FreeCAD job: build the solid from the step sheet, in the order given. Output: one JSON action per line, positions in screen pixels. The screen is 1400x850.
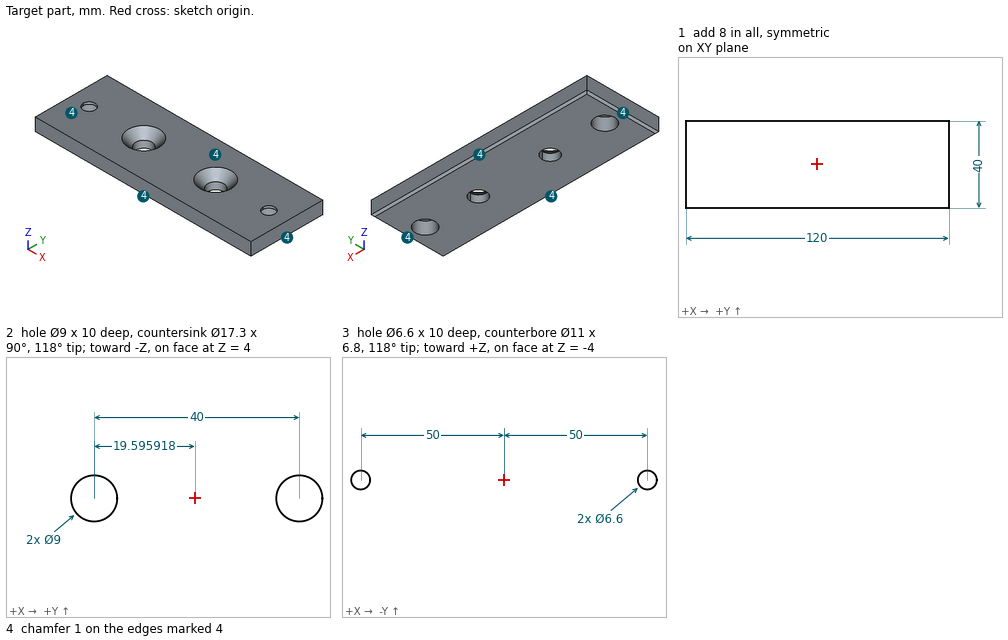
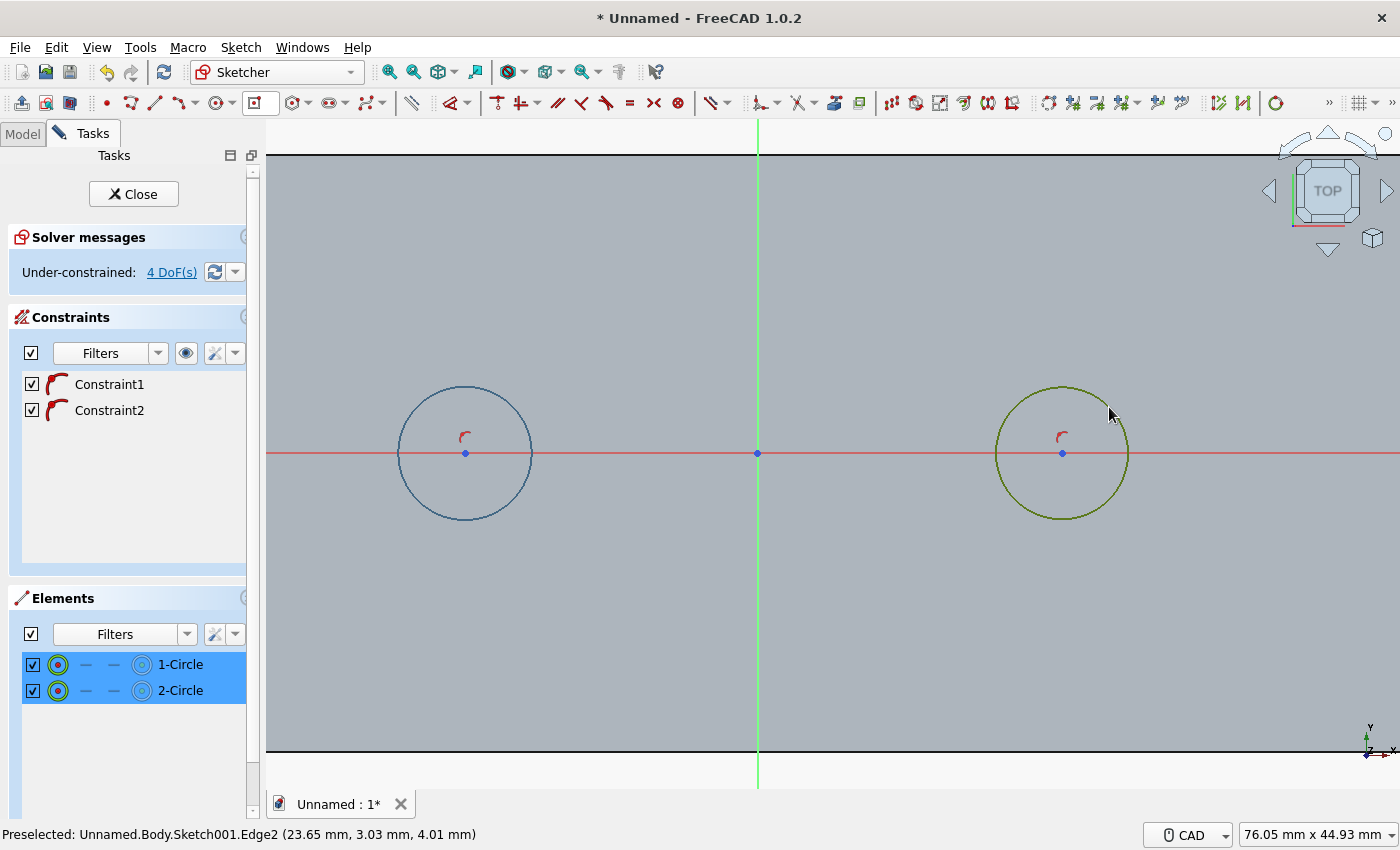
{"action": "key", "text": "e"}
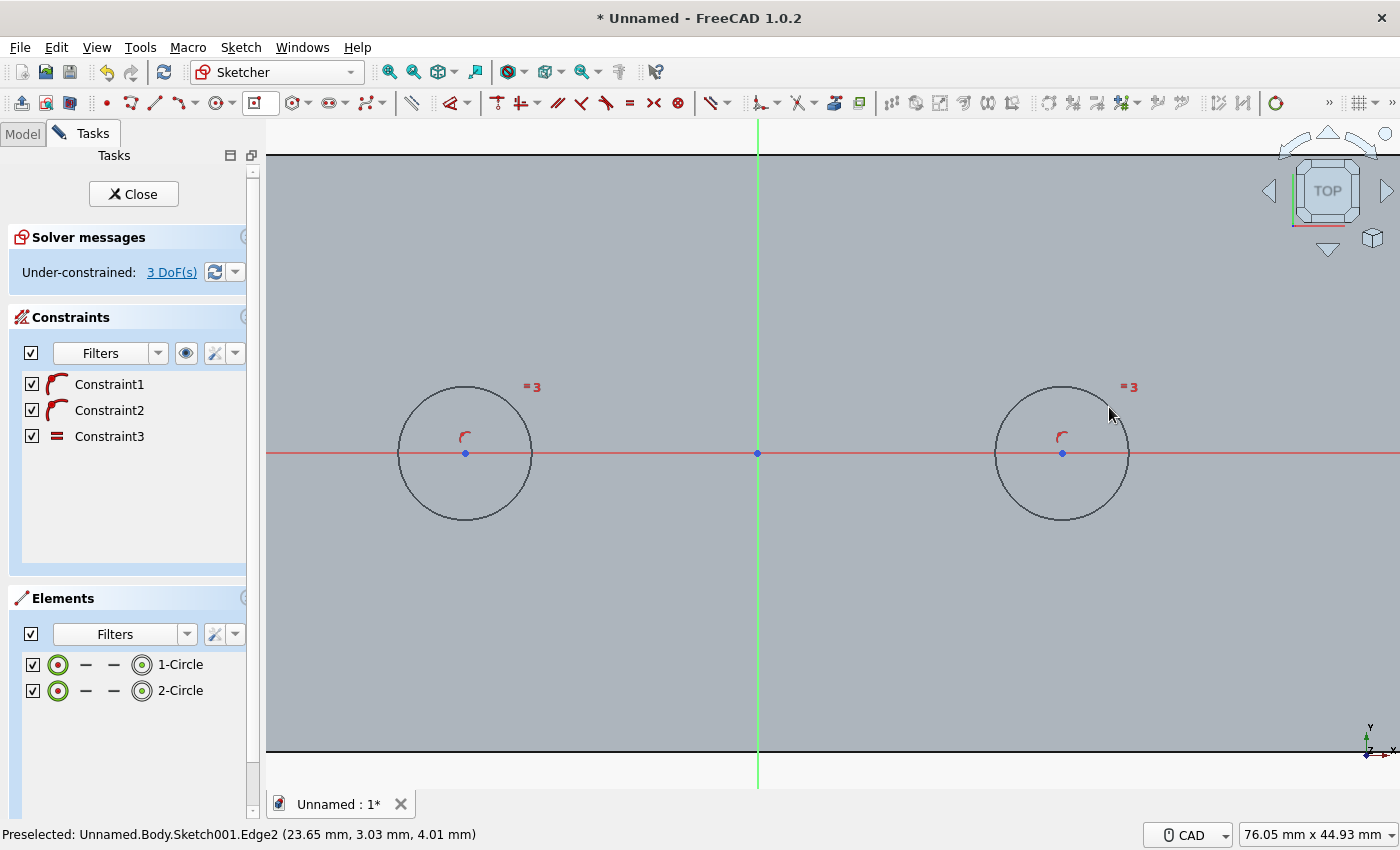
{"action": "left_click", "coordinate": [512, 406]}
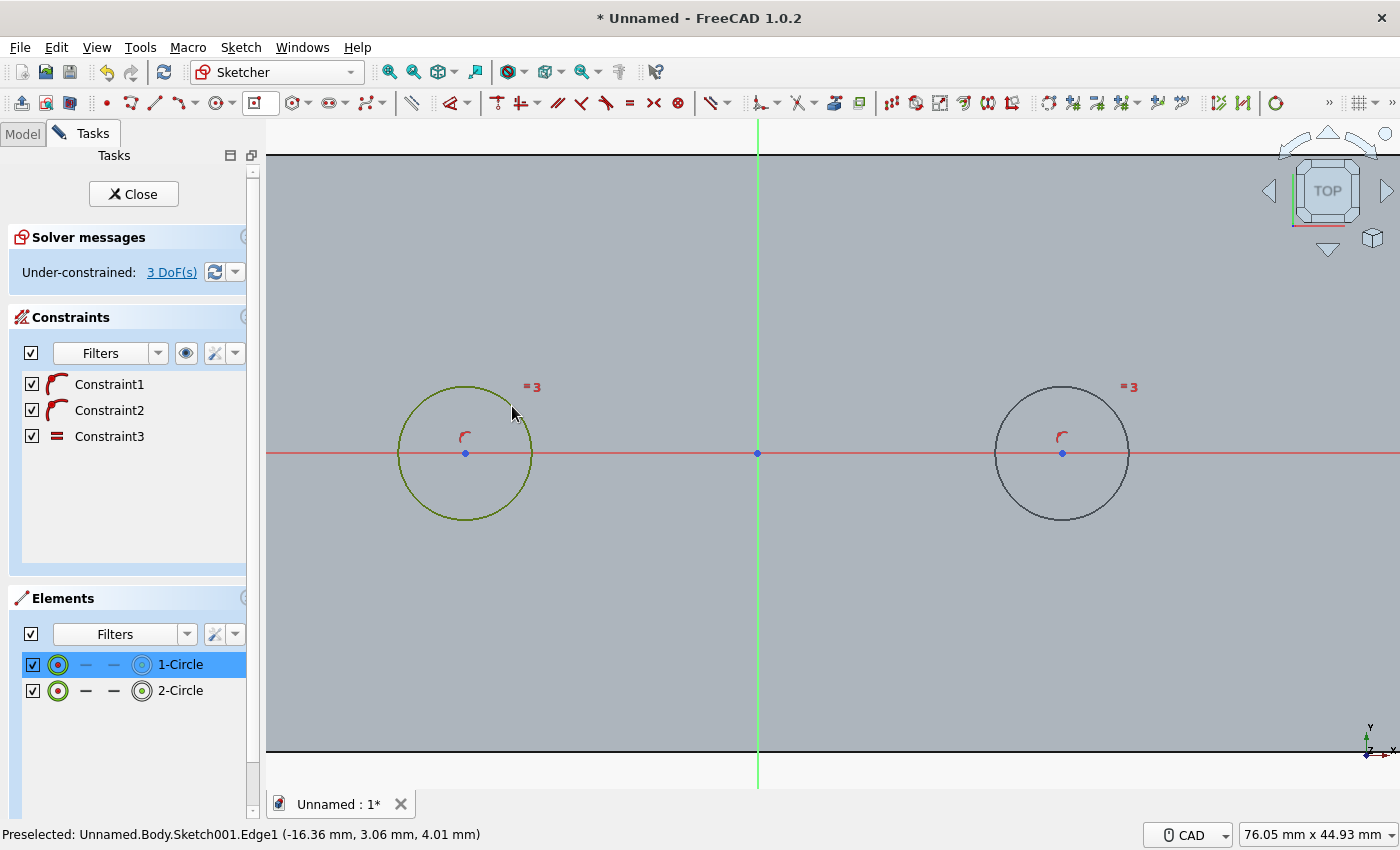
{"action": "key", "text": "k o"}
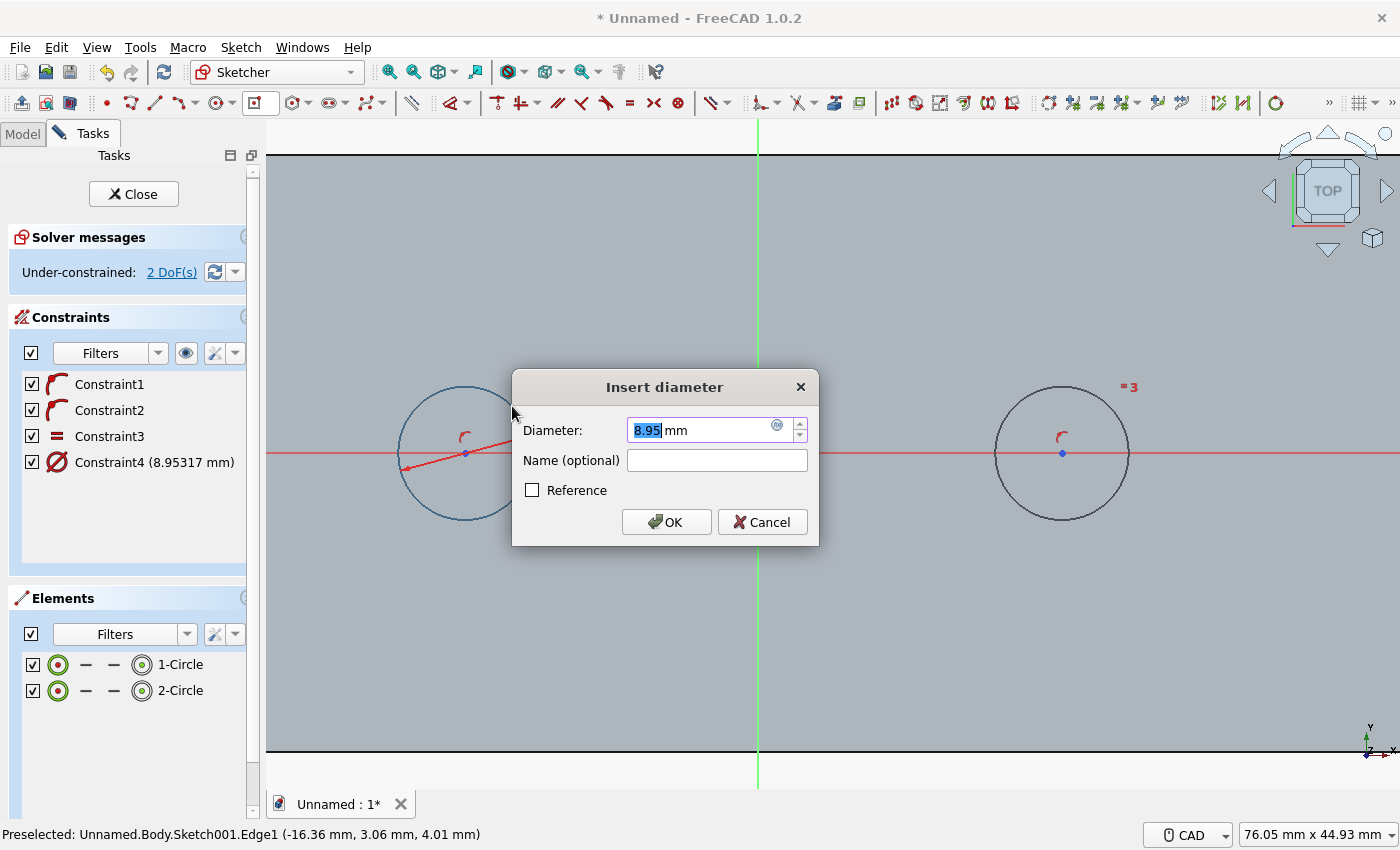
{"action": "type", "text": "9"}
{"action": "key", "text": "Return"}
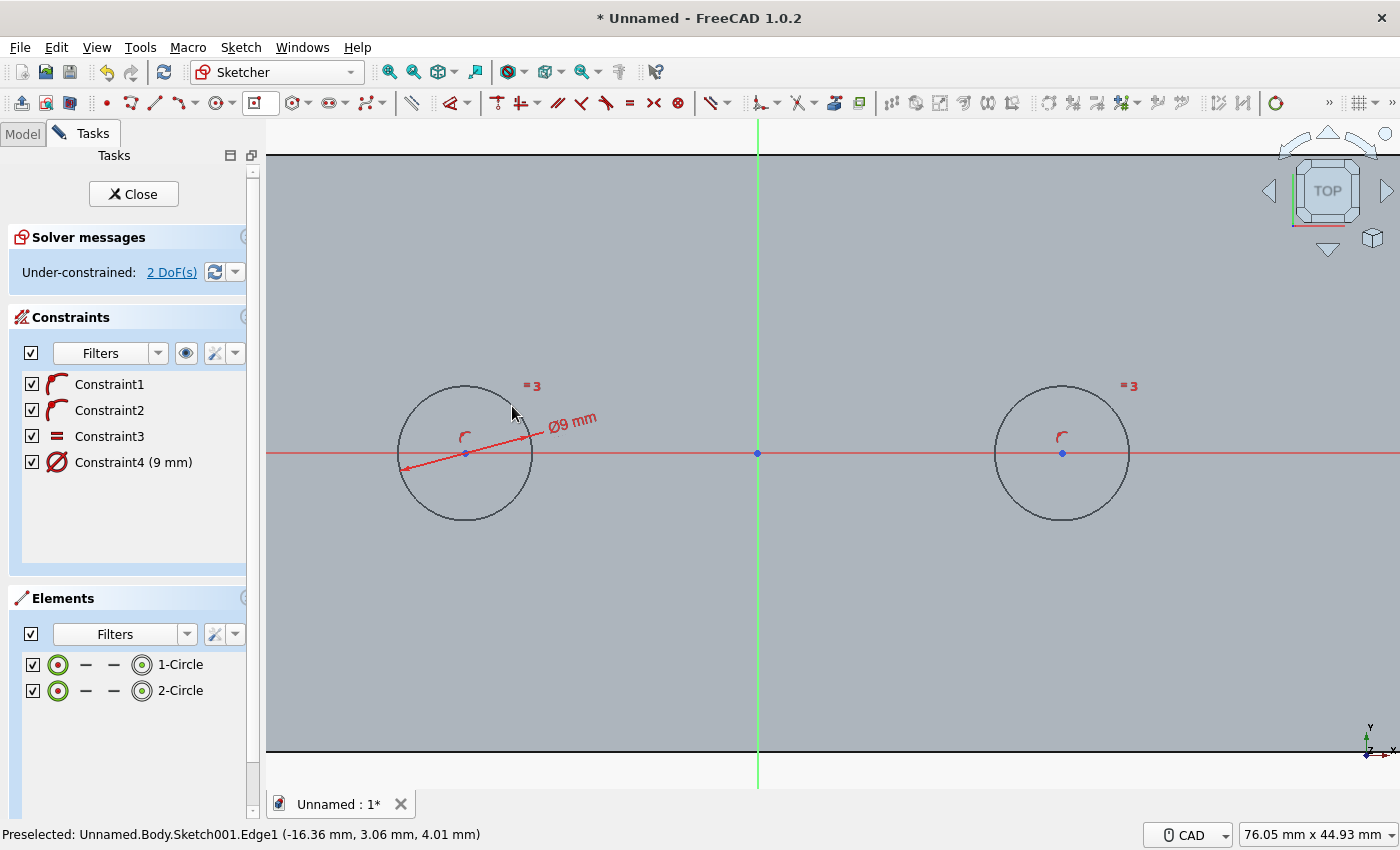
{"action": "left_click", "coordinate": [465, 453]}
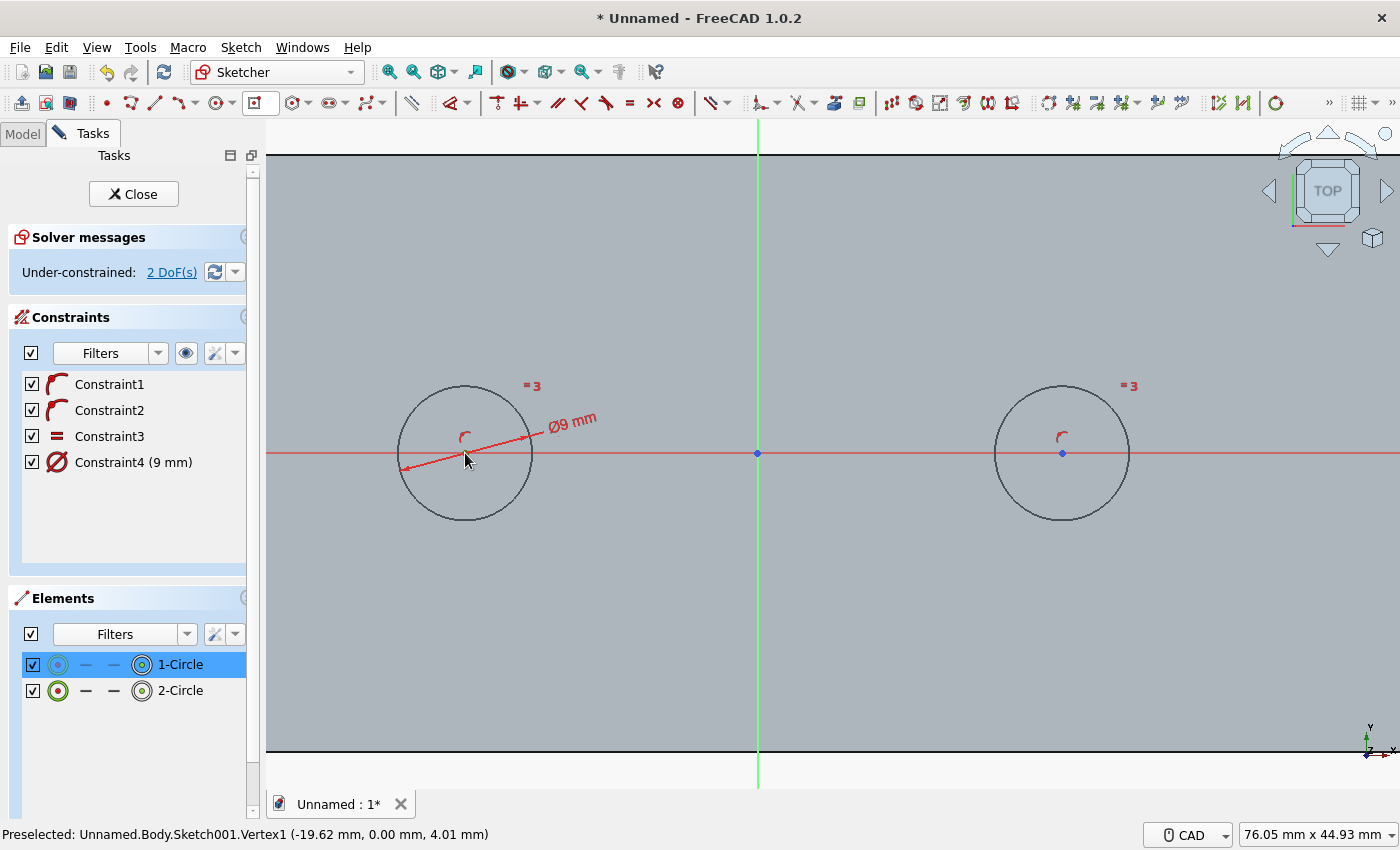
{"action": "left_click", "coordinate": [1062, 453]}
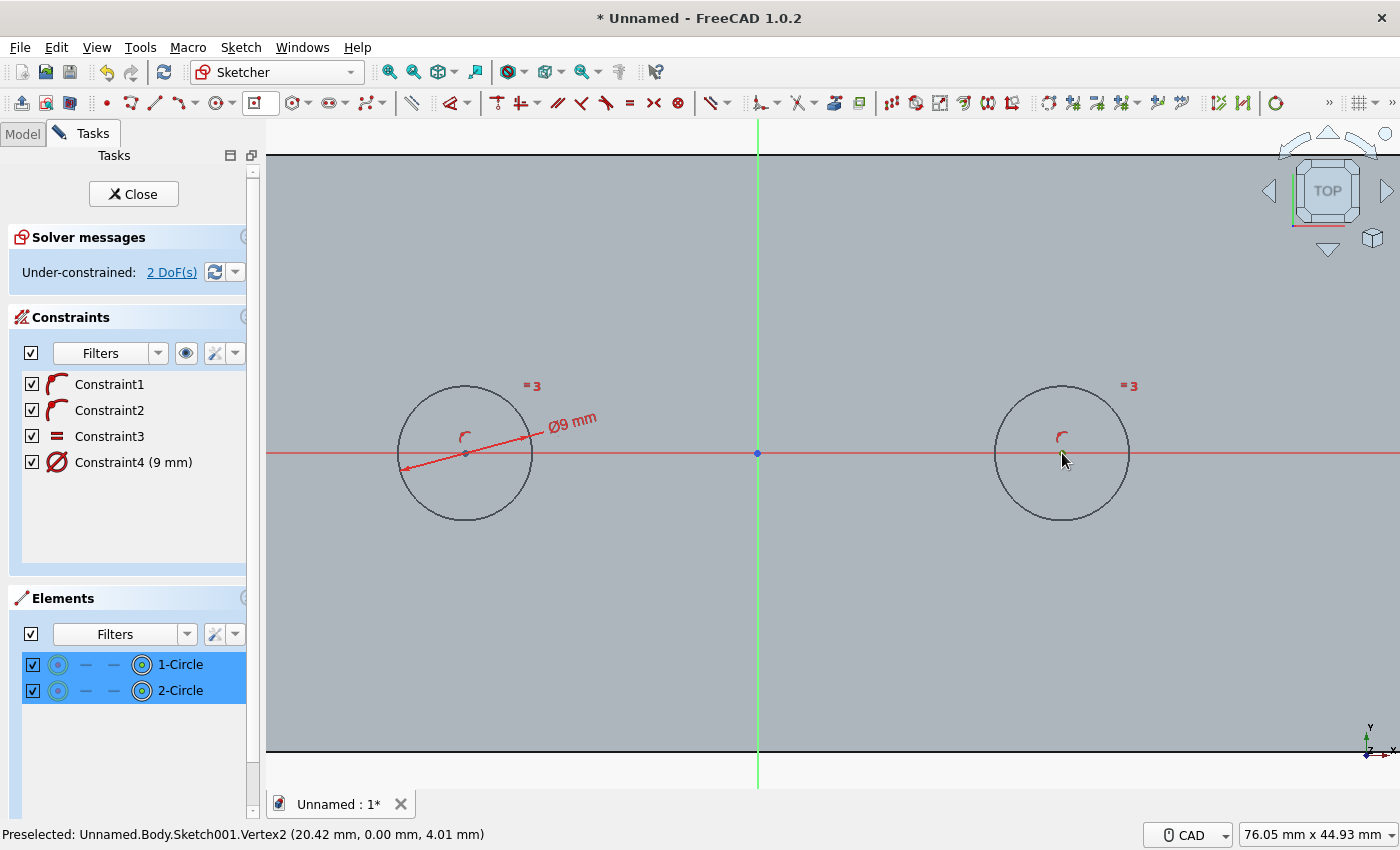
{"action": "key", "text": "l"}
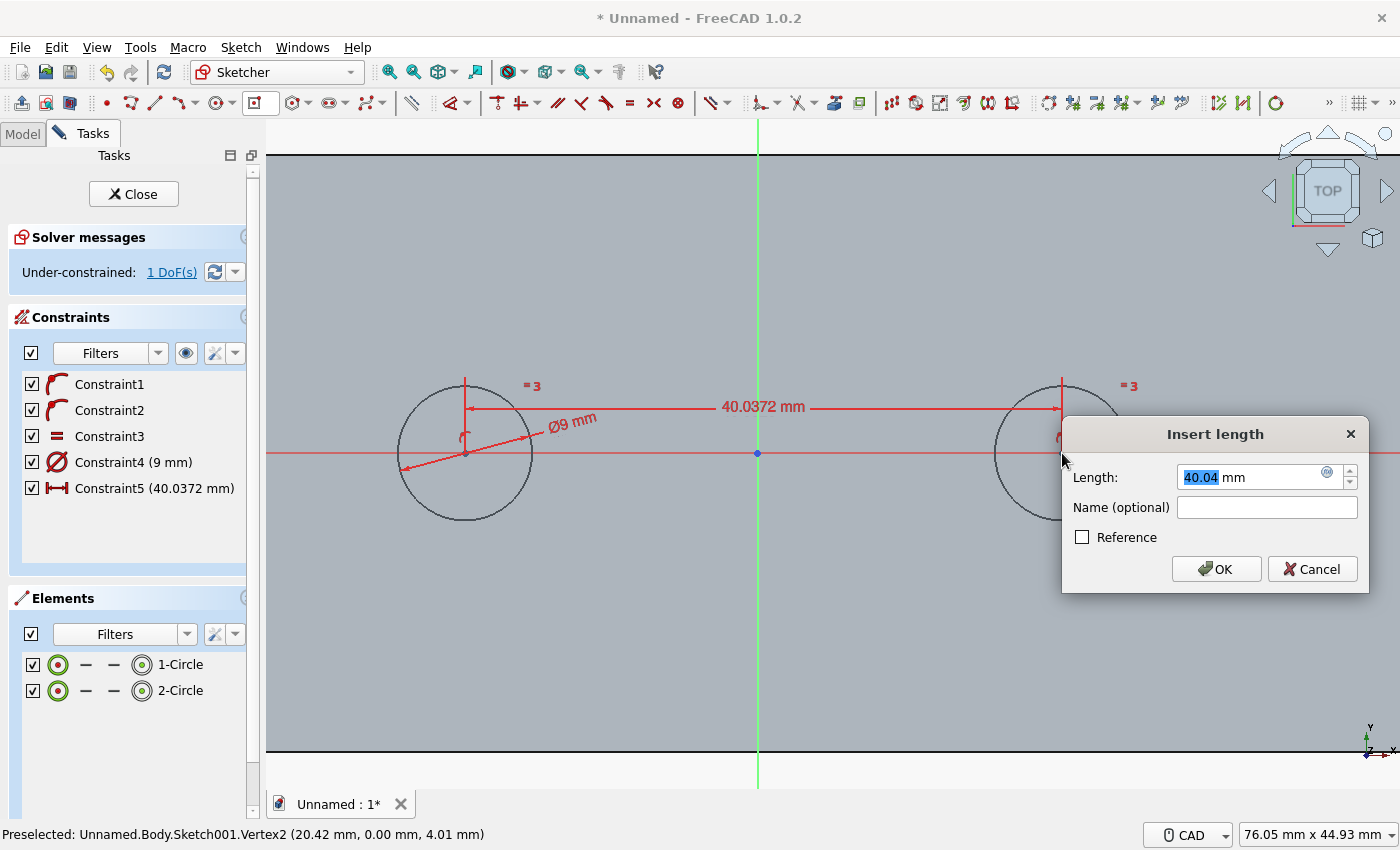
{"action": "type", "text": "40"}
{"action": "key", "text": "Return"}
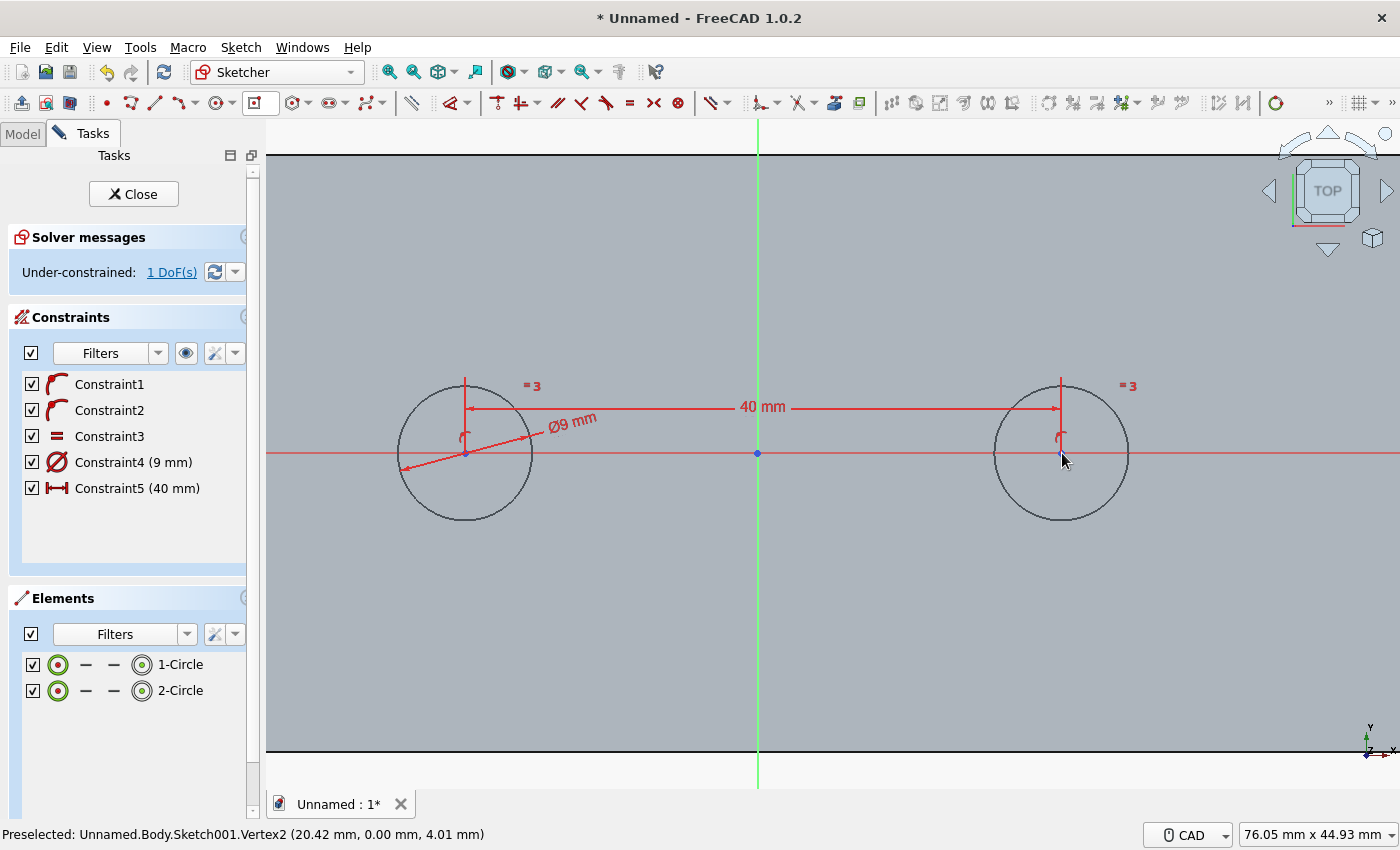
{"action": "left_click", "coordinate": [465, 453]}